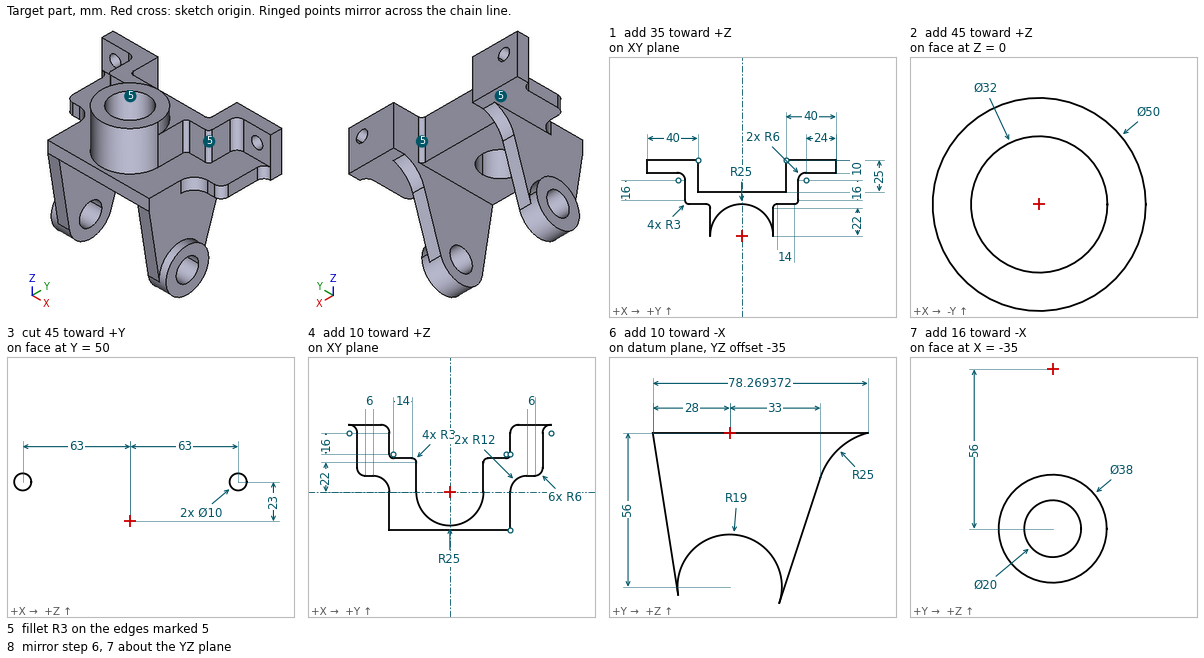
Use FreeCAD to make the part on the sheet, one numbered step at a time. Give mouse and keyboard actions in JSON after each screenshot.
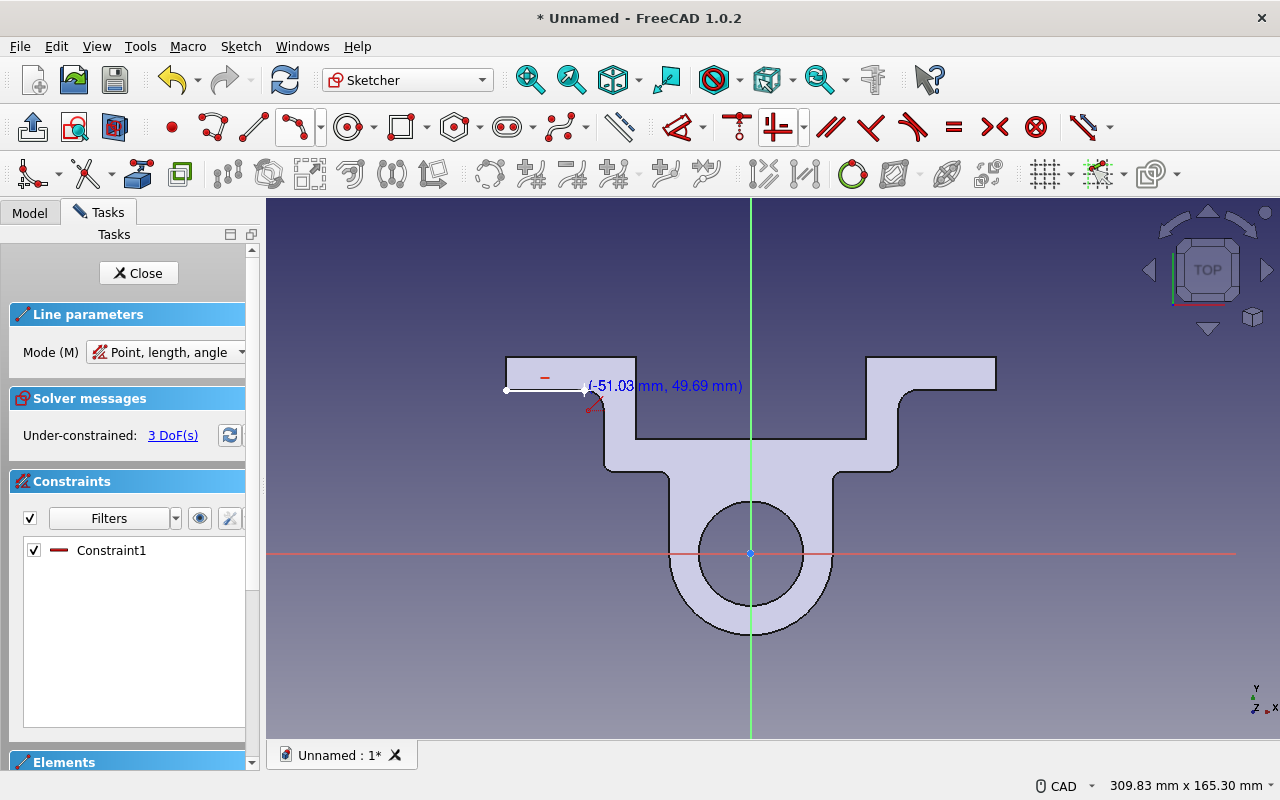
{"action": "left_click", "coordinate": [604, 410]}
{"action": "left_click", "coordinate": [604, 462]}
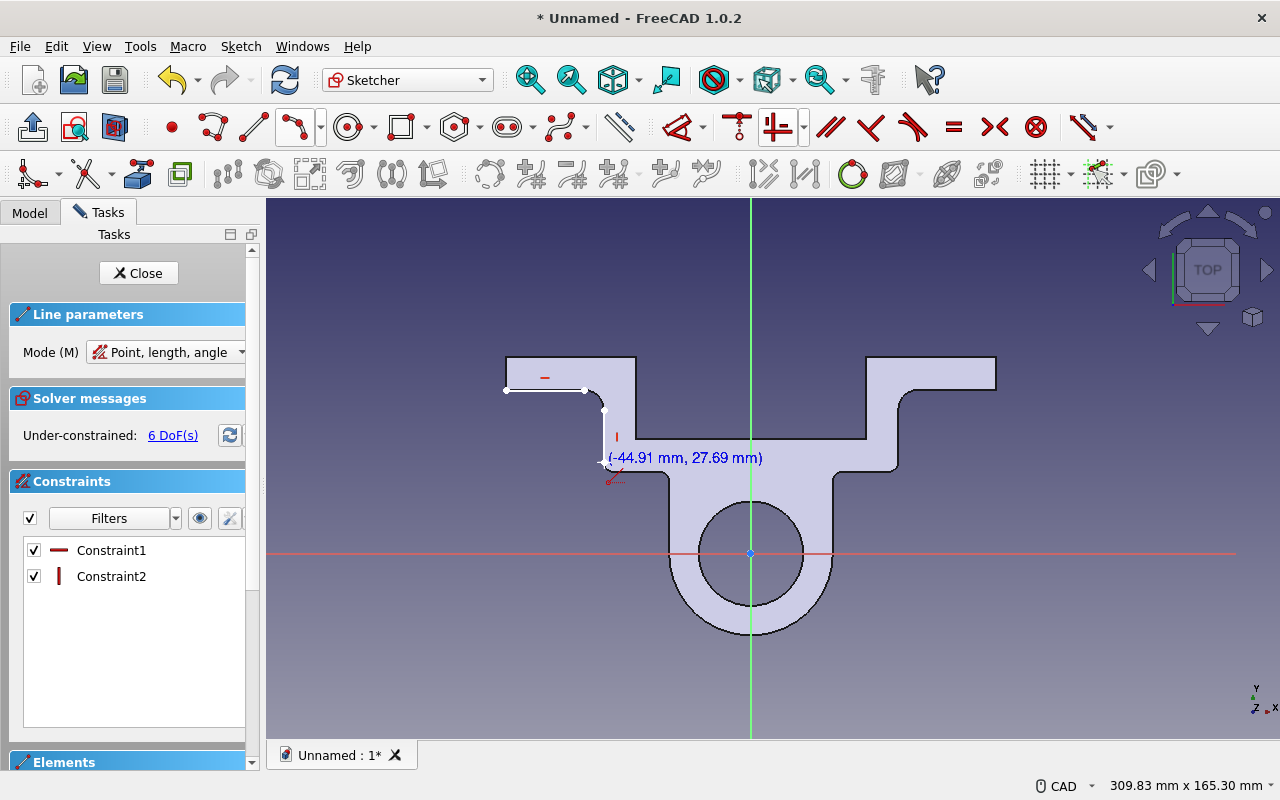
{"action": "left_click", "coordinate": [614, 472]}
{"action": "left_click", "coordinate": [659, 472]}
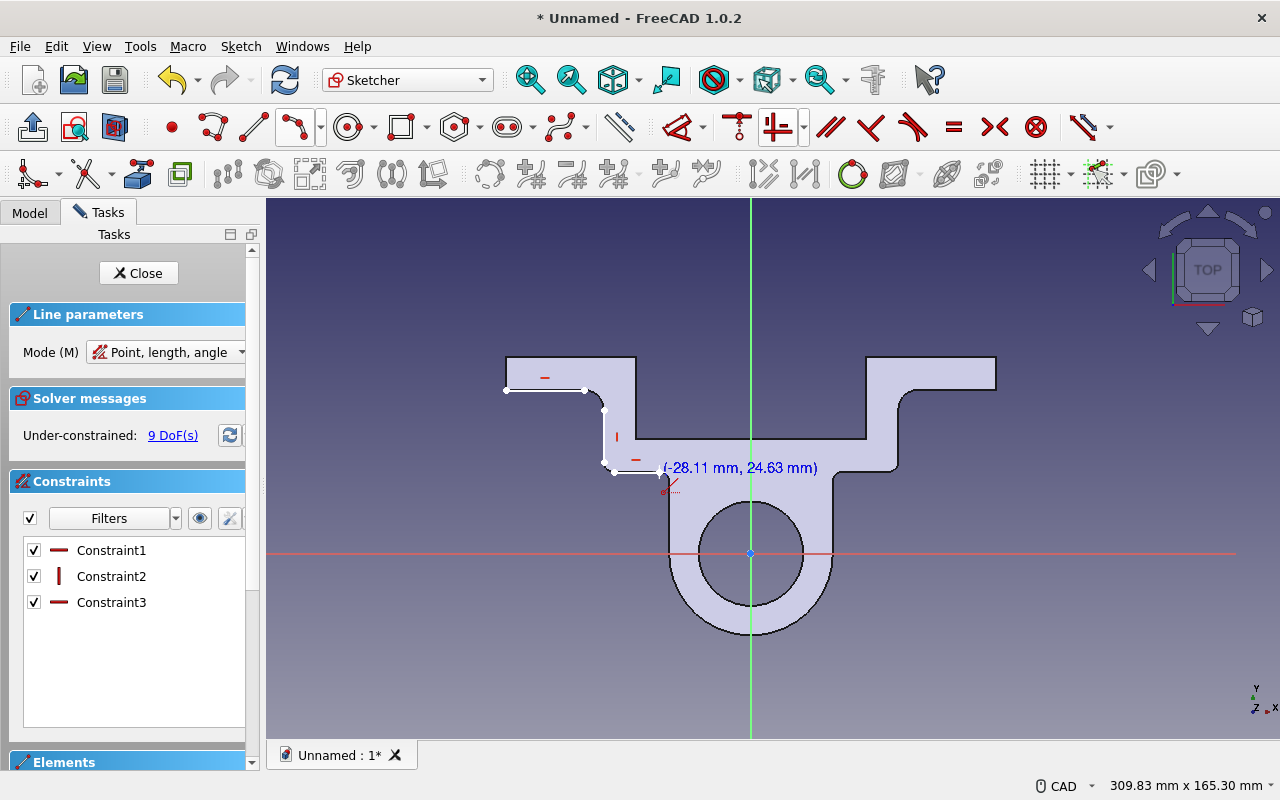
{"action": "left_click", "coordinate": [669, 482]}
{"action": "left_click", "coordinate": [669, 554]}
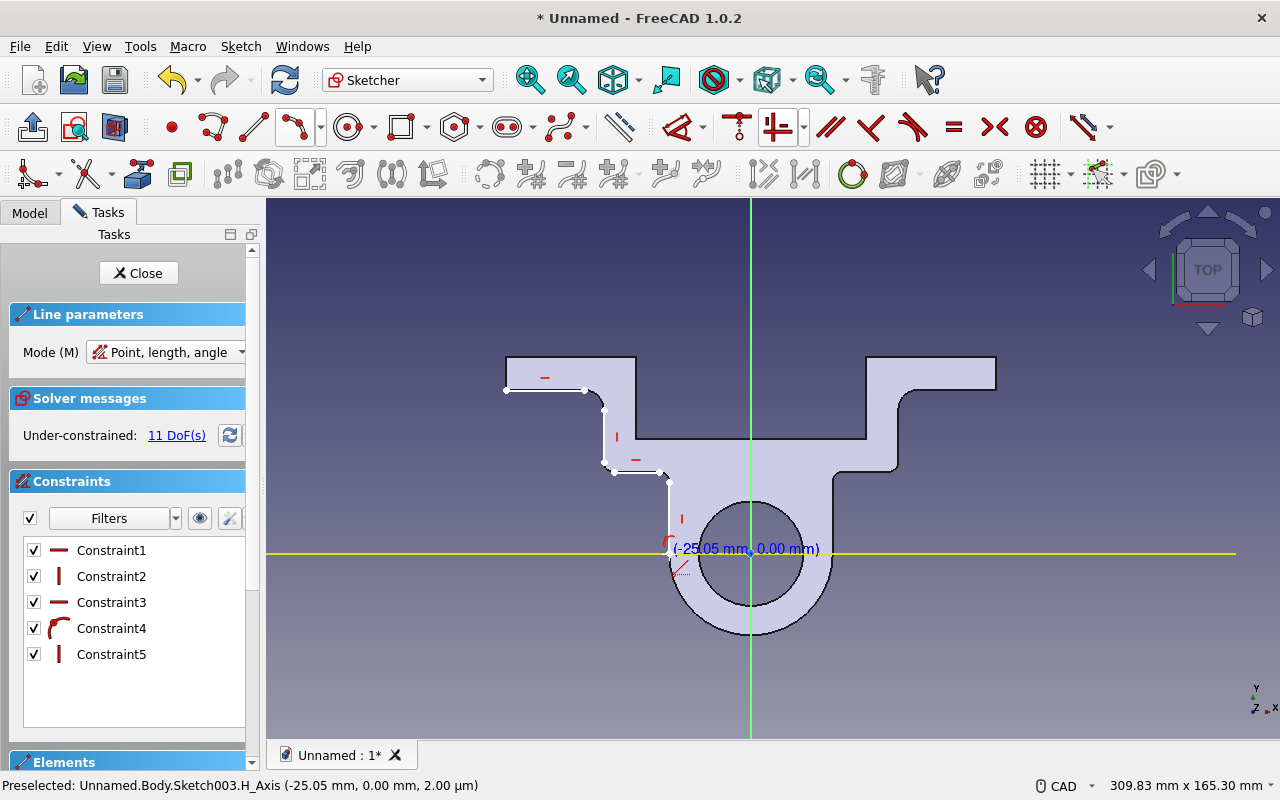
{"action": "left_click", "coordinate": [833, 554]}
{"action": "left_click", "coordinate": [833, 482]}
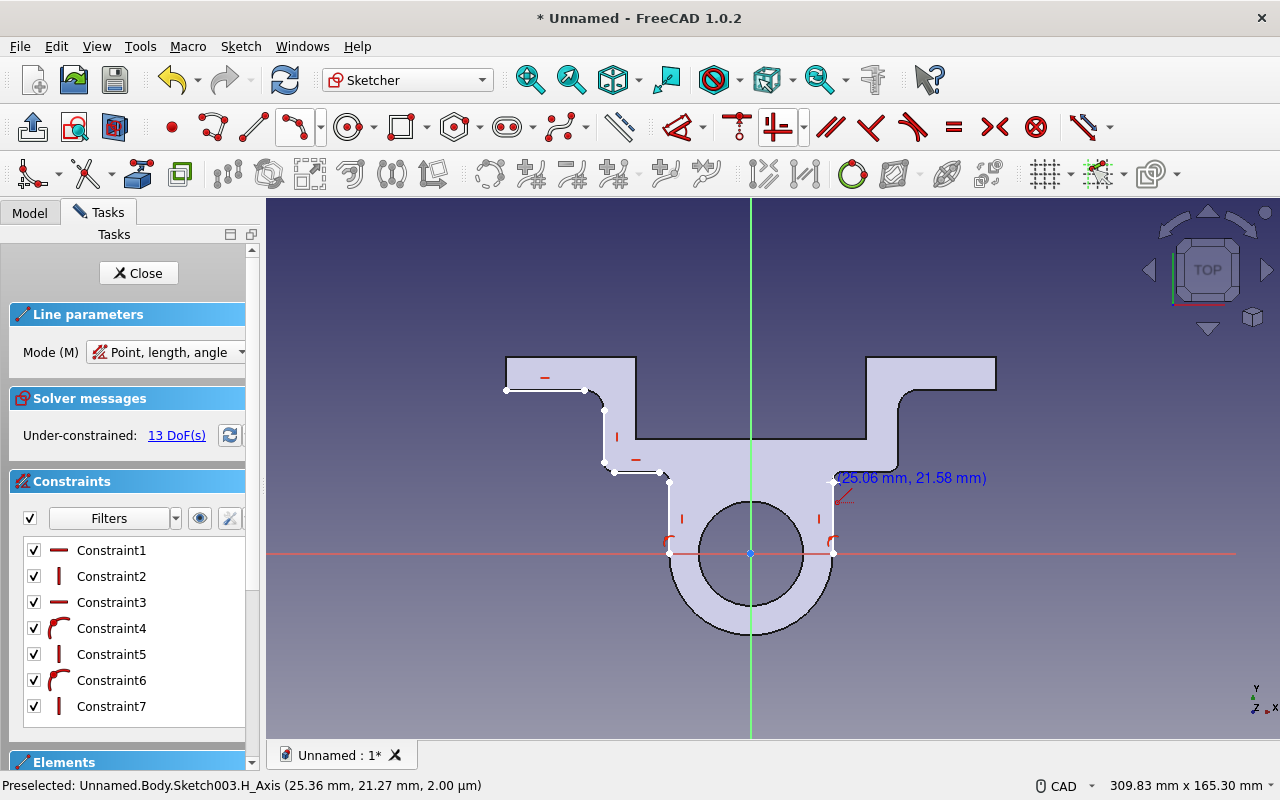
{"action": "left_click", "coordinate": [843, 472]}
{"action": "left_click", "coordinate": [888, 472]}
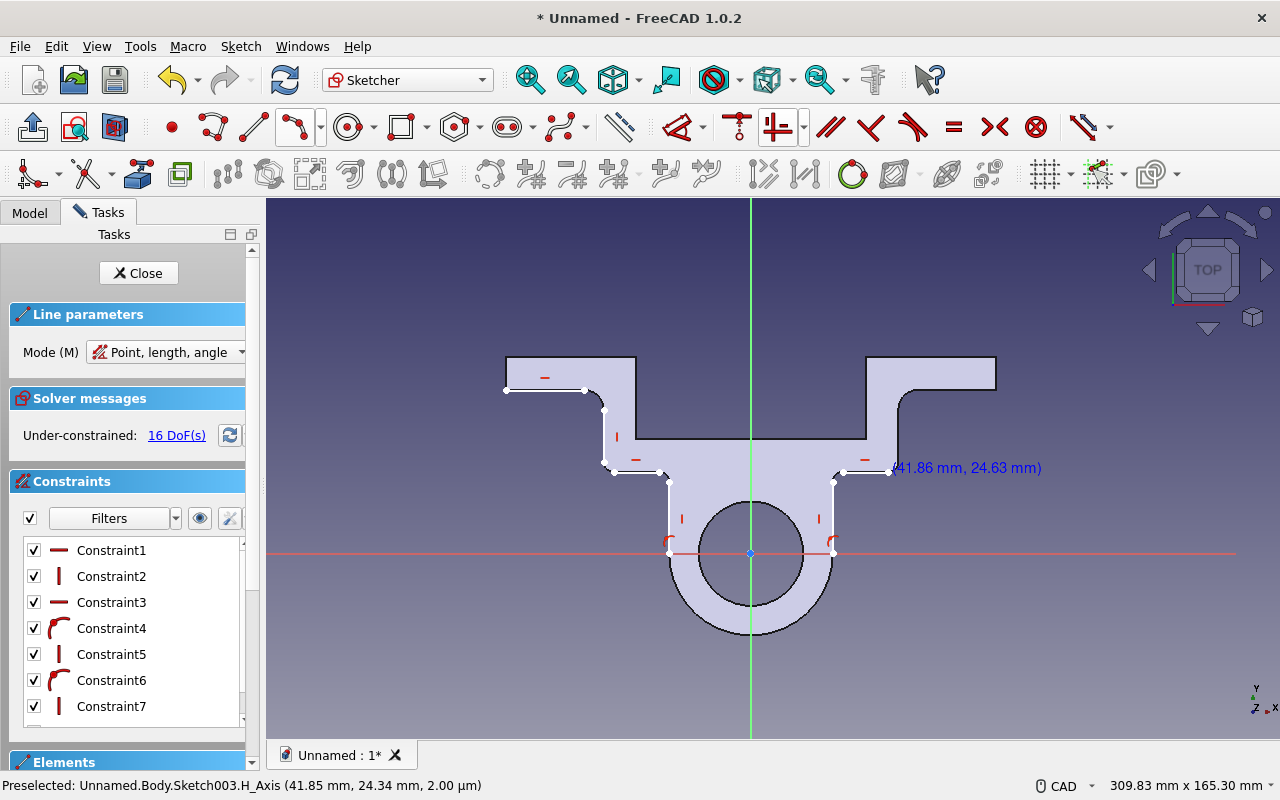
{"action": "left_click", "coordinate": [898, 462]}
{"action": "left_click", "coordinate": [898, 410]}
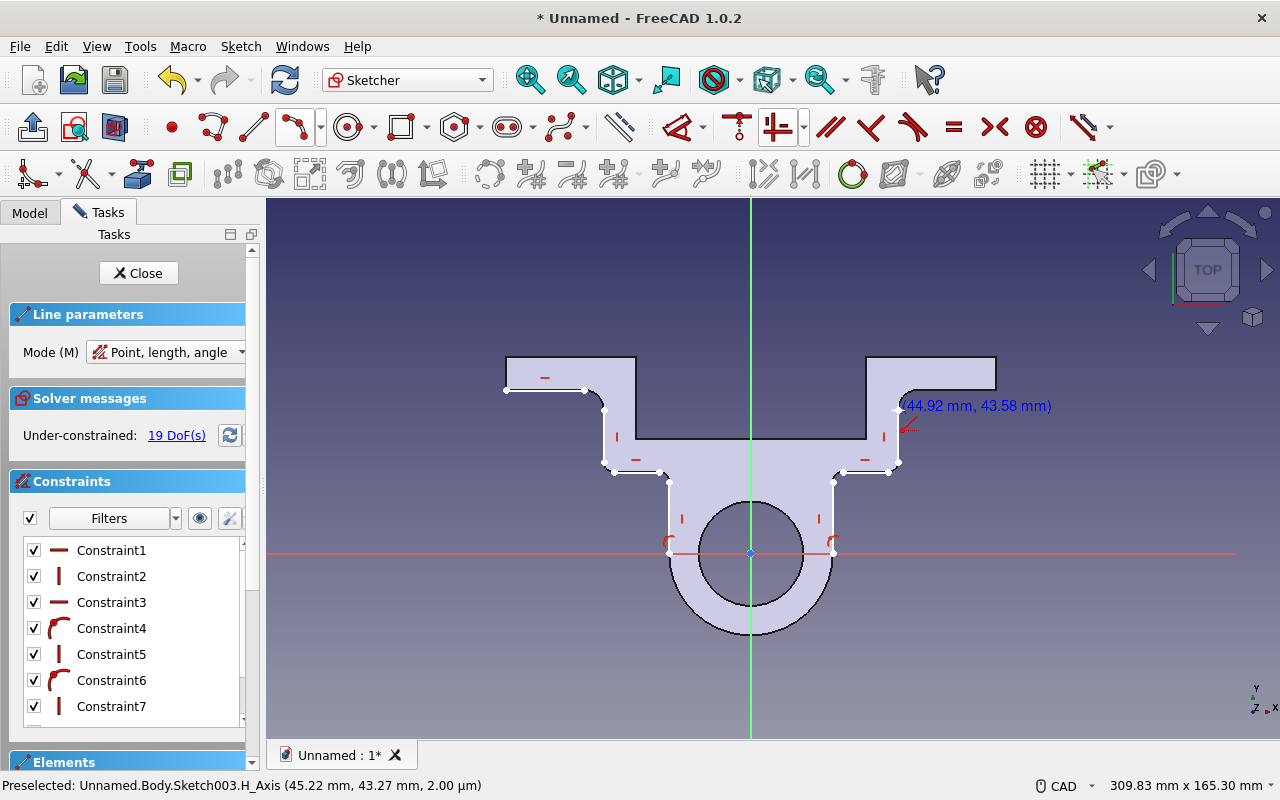
{"action": "left_click", "coordinate": [918, 390]}
{"action": "left_click", "coordinate": [996, 390]}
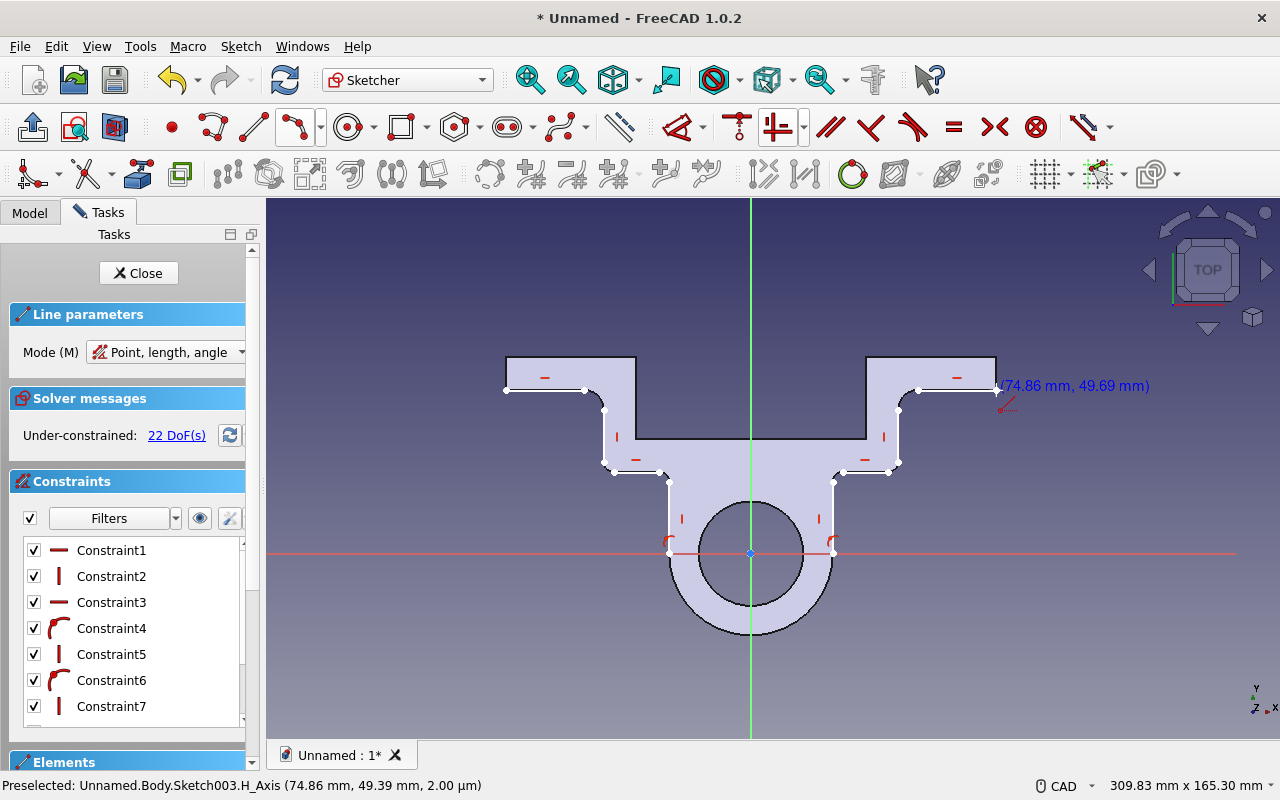
{"action": "left_click", "coordinate": [977, 410]}
{"action": "left_click", "coordinate": [977, 495]}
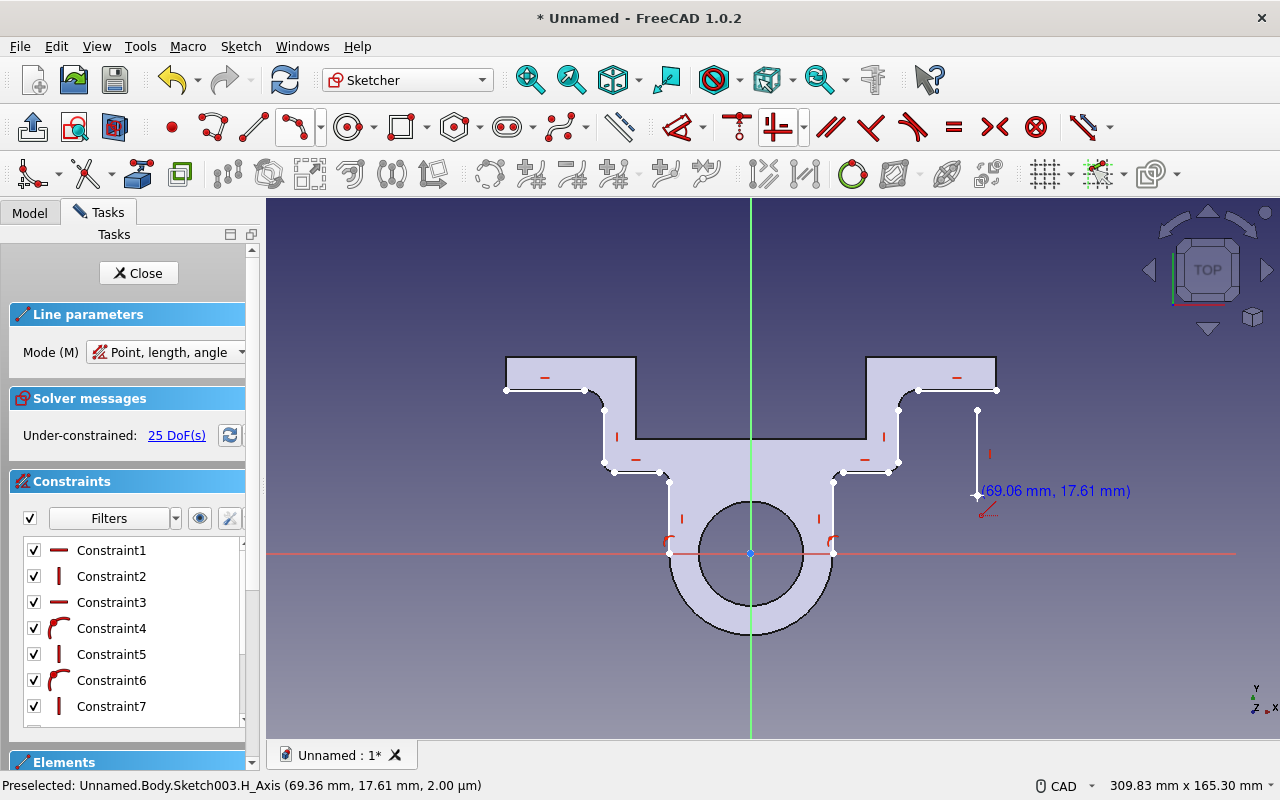
{"action": "left_click", "coordinate": [957, 514]}
{"action": "left_click", "coordinate": [938, 514]}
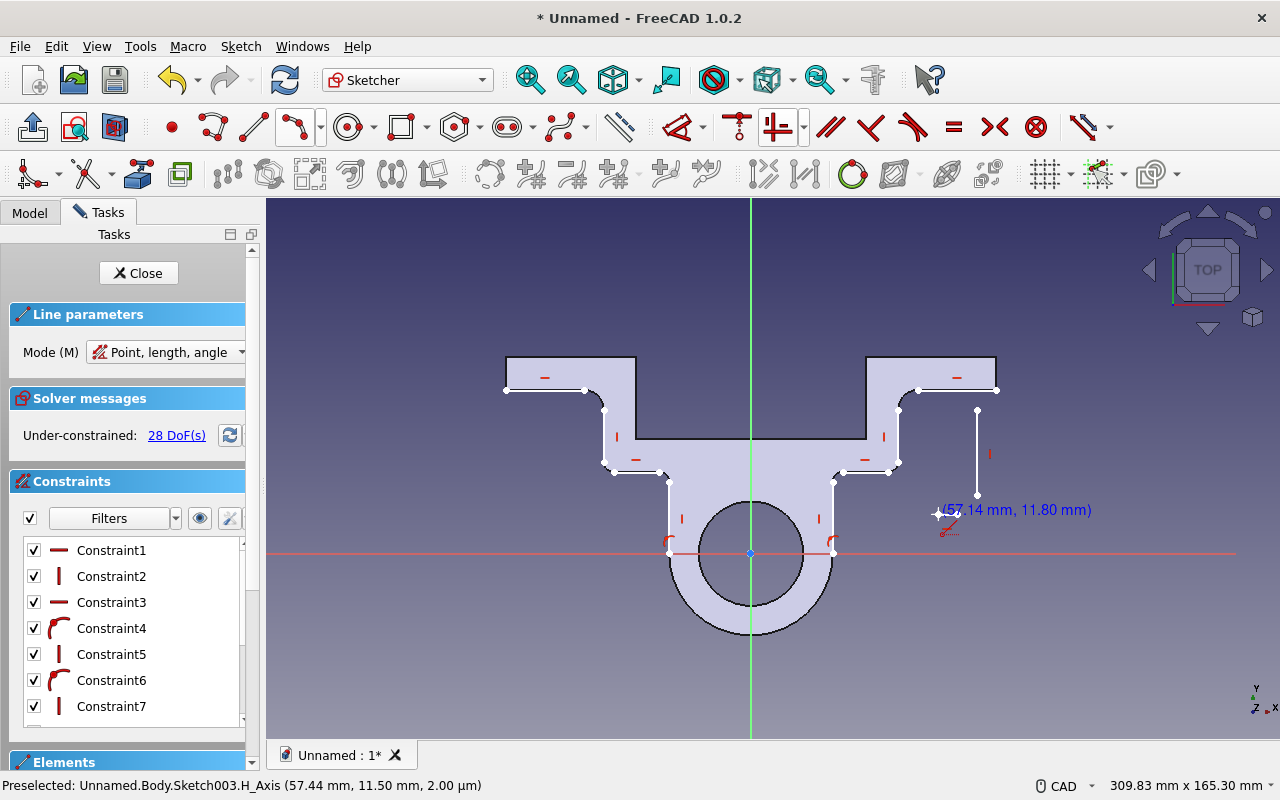
{"action": "left_click", "coordinate": [213, 128]}